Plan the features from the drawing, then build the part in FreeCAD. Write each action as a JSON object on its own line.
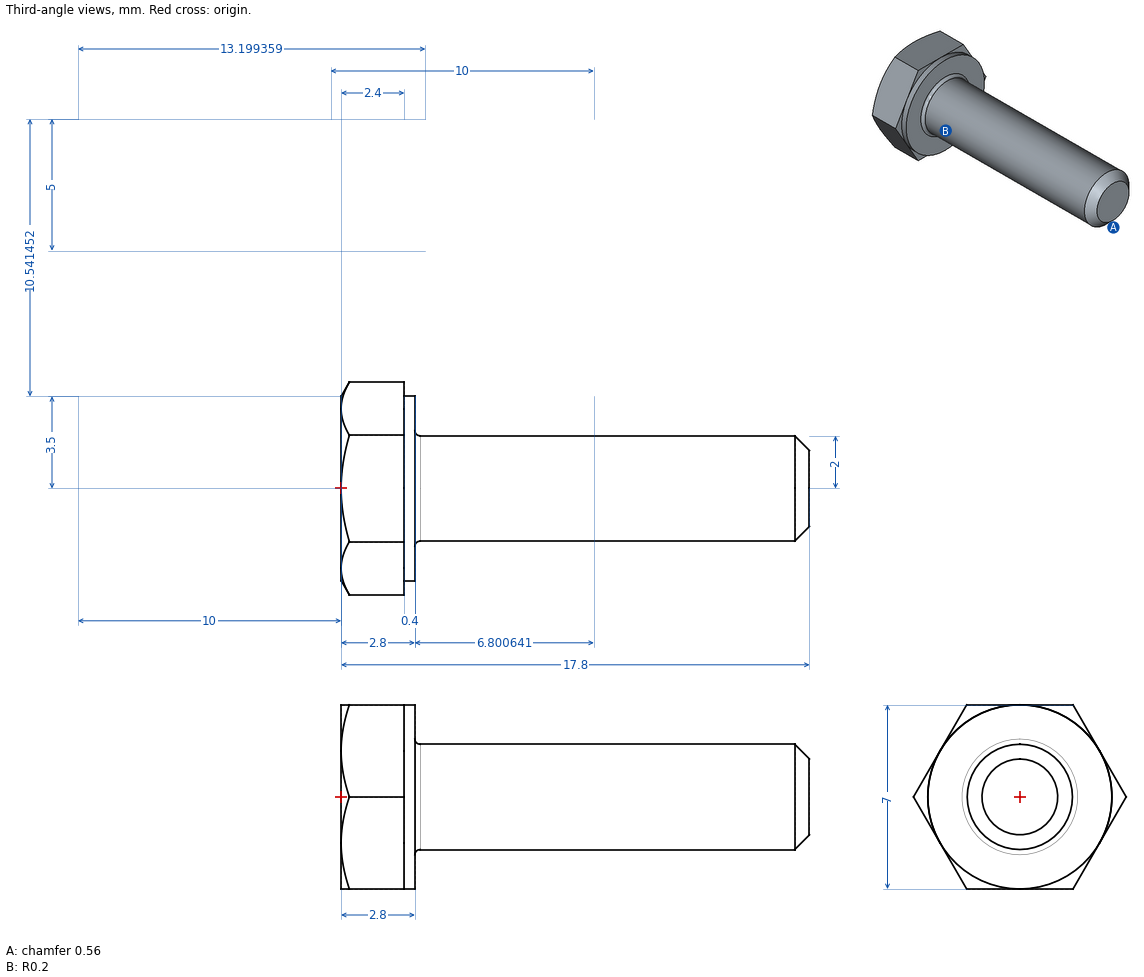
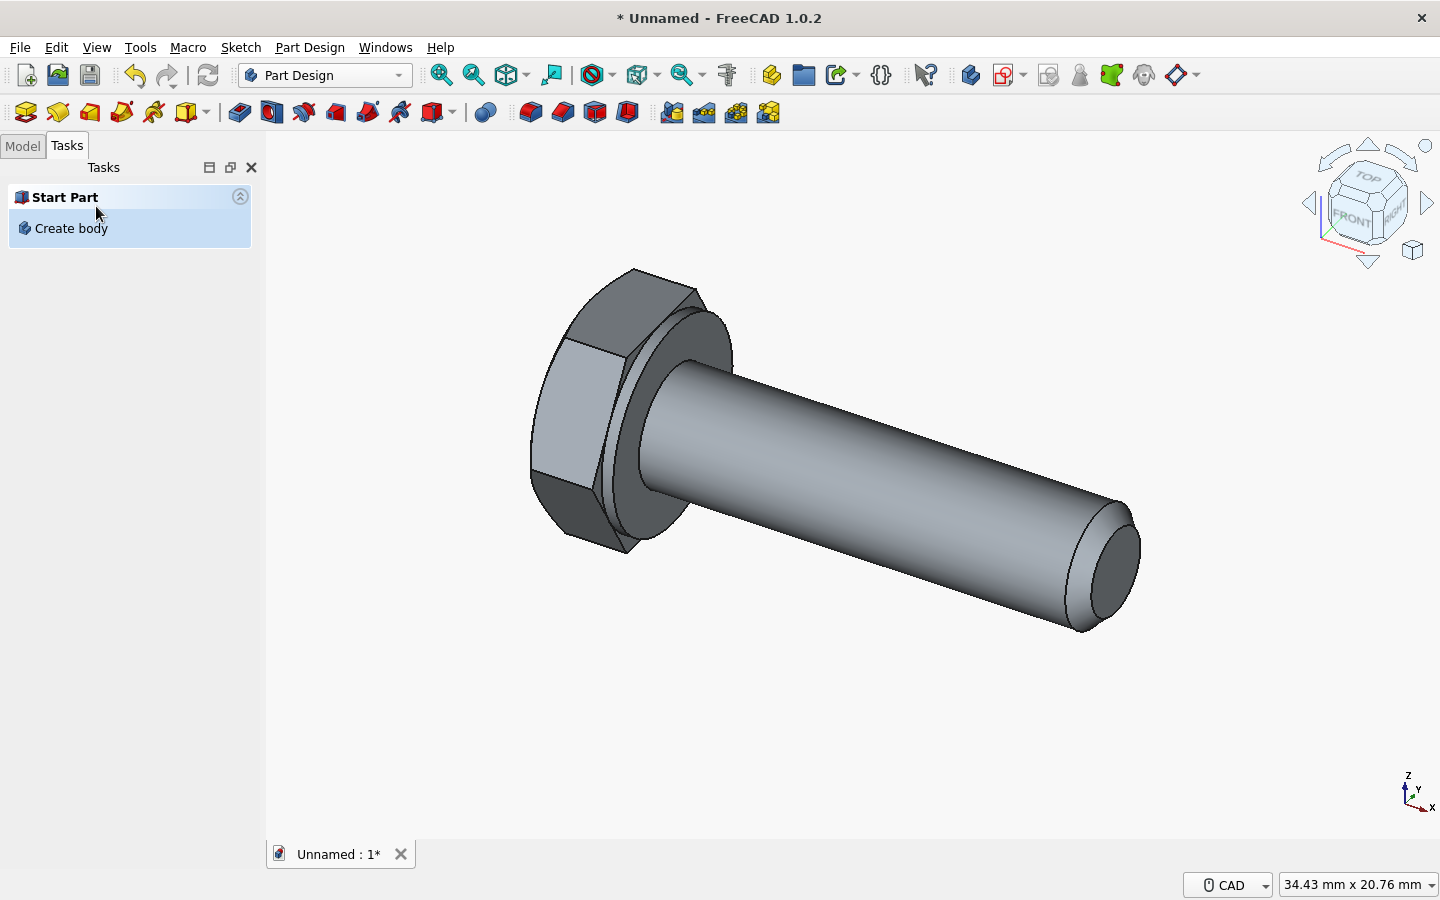
{"action": "key", "text": "0"}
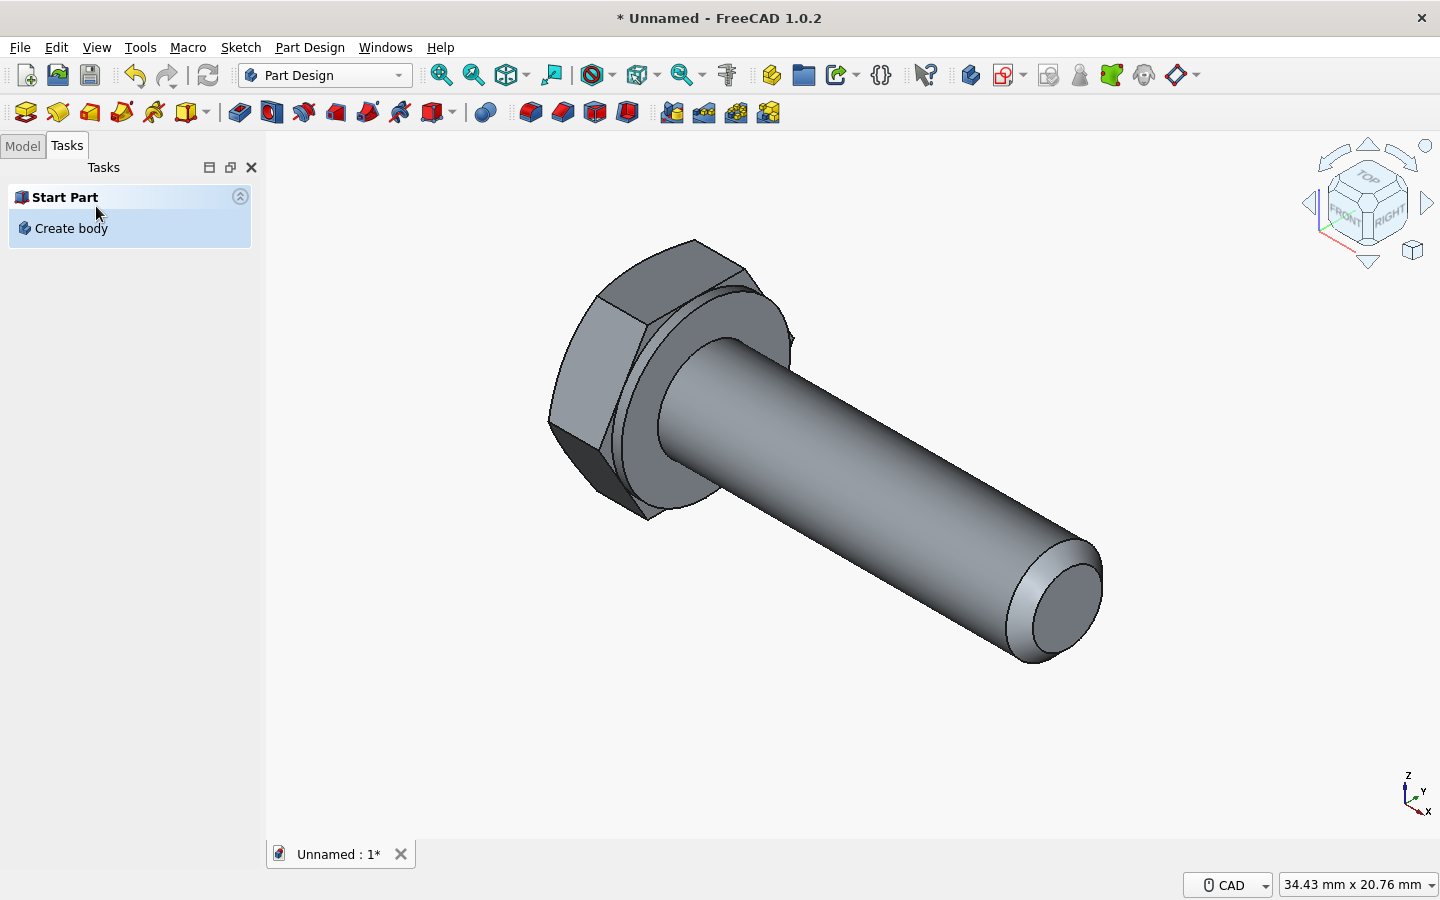
{"action": "key", "text": "2"}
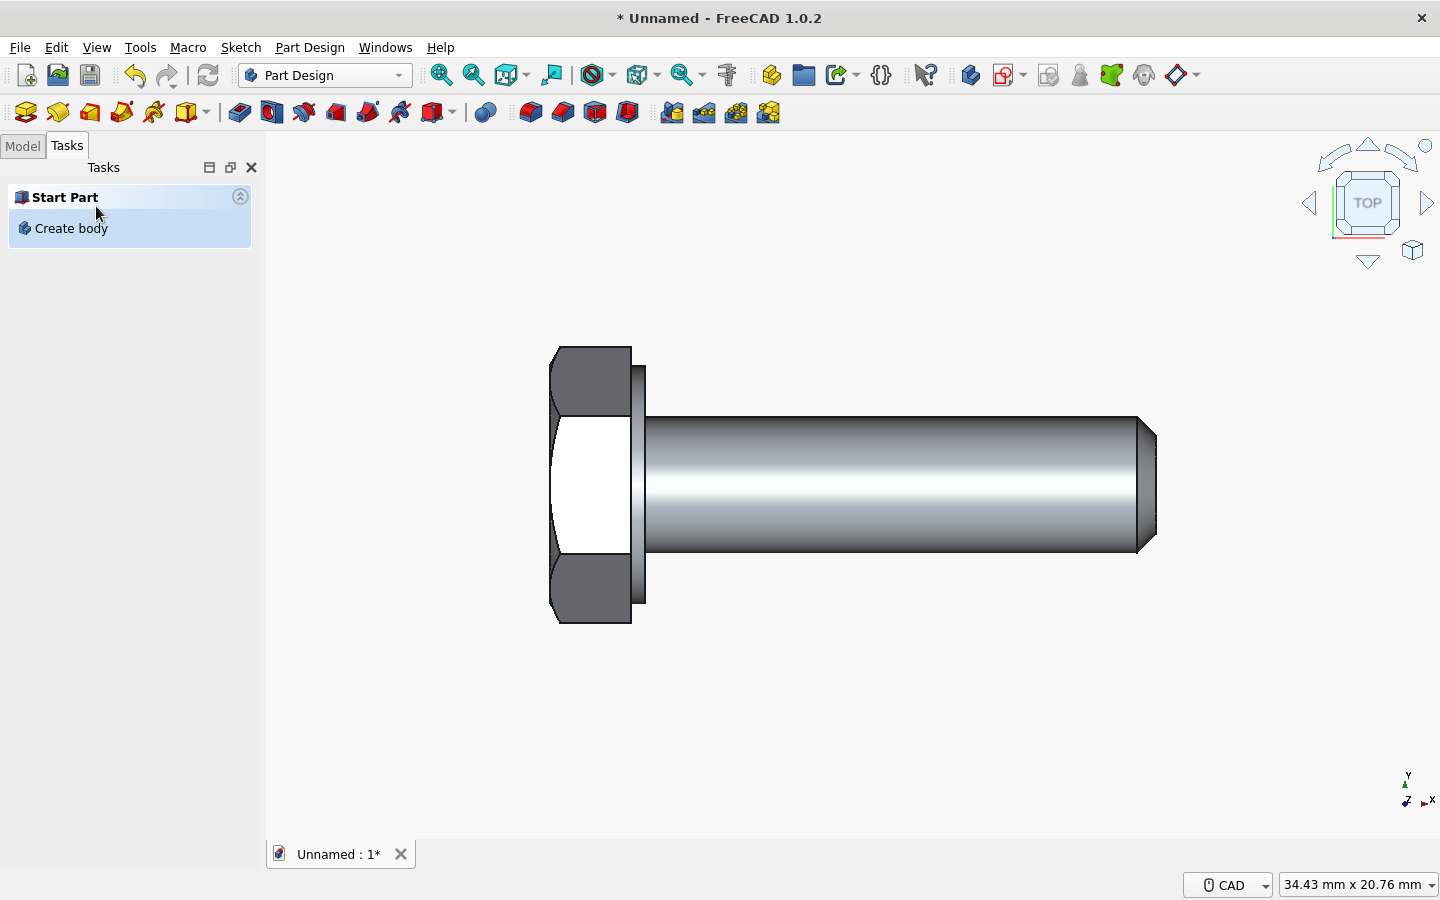
{"action": "key", "text": "1"}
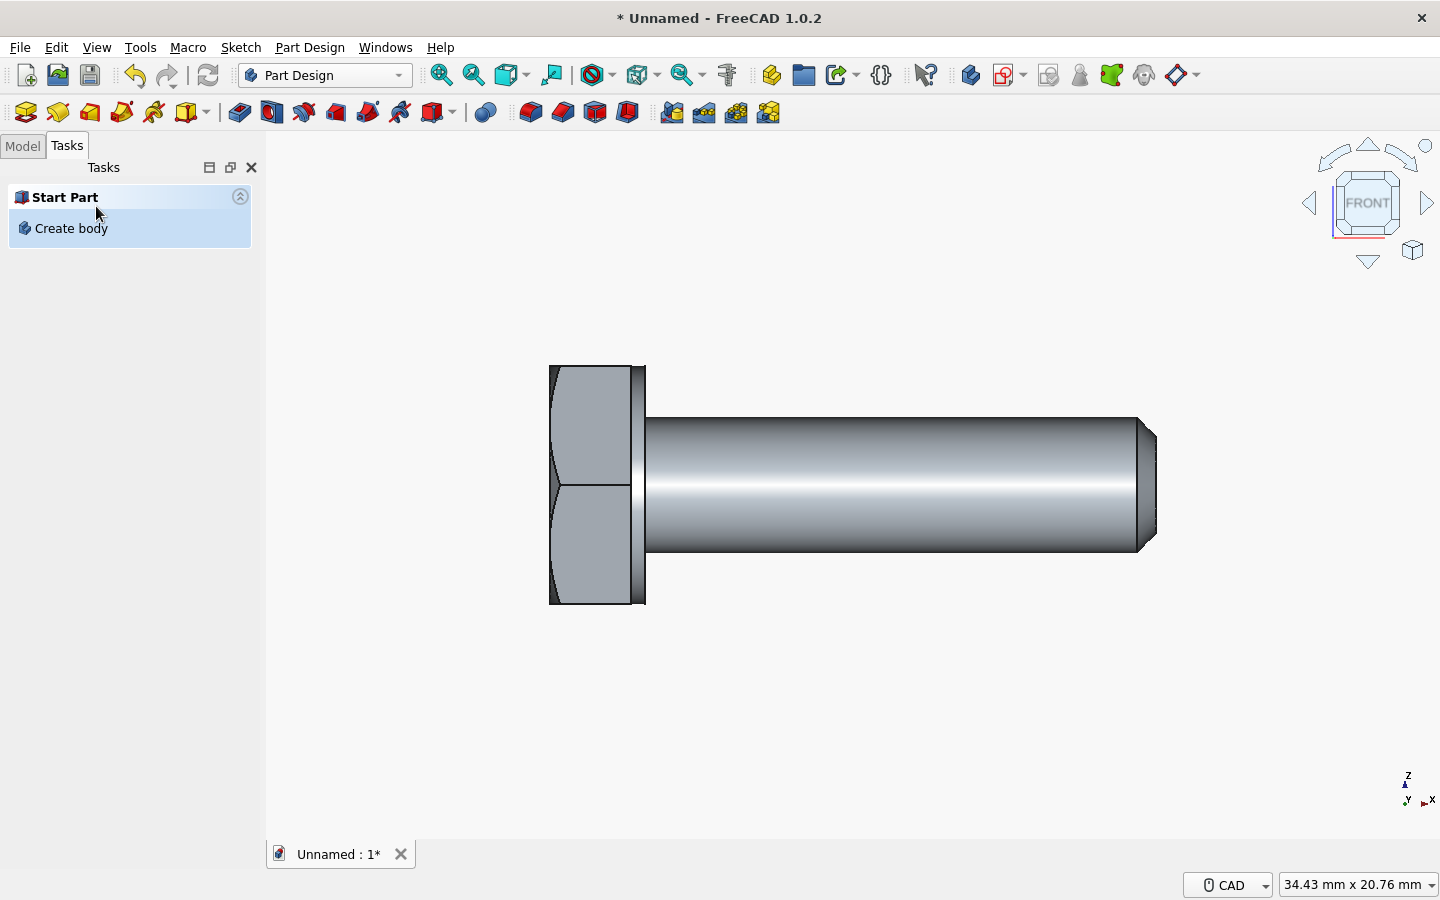
{"action": "key", "text": "3"}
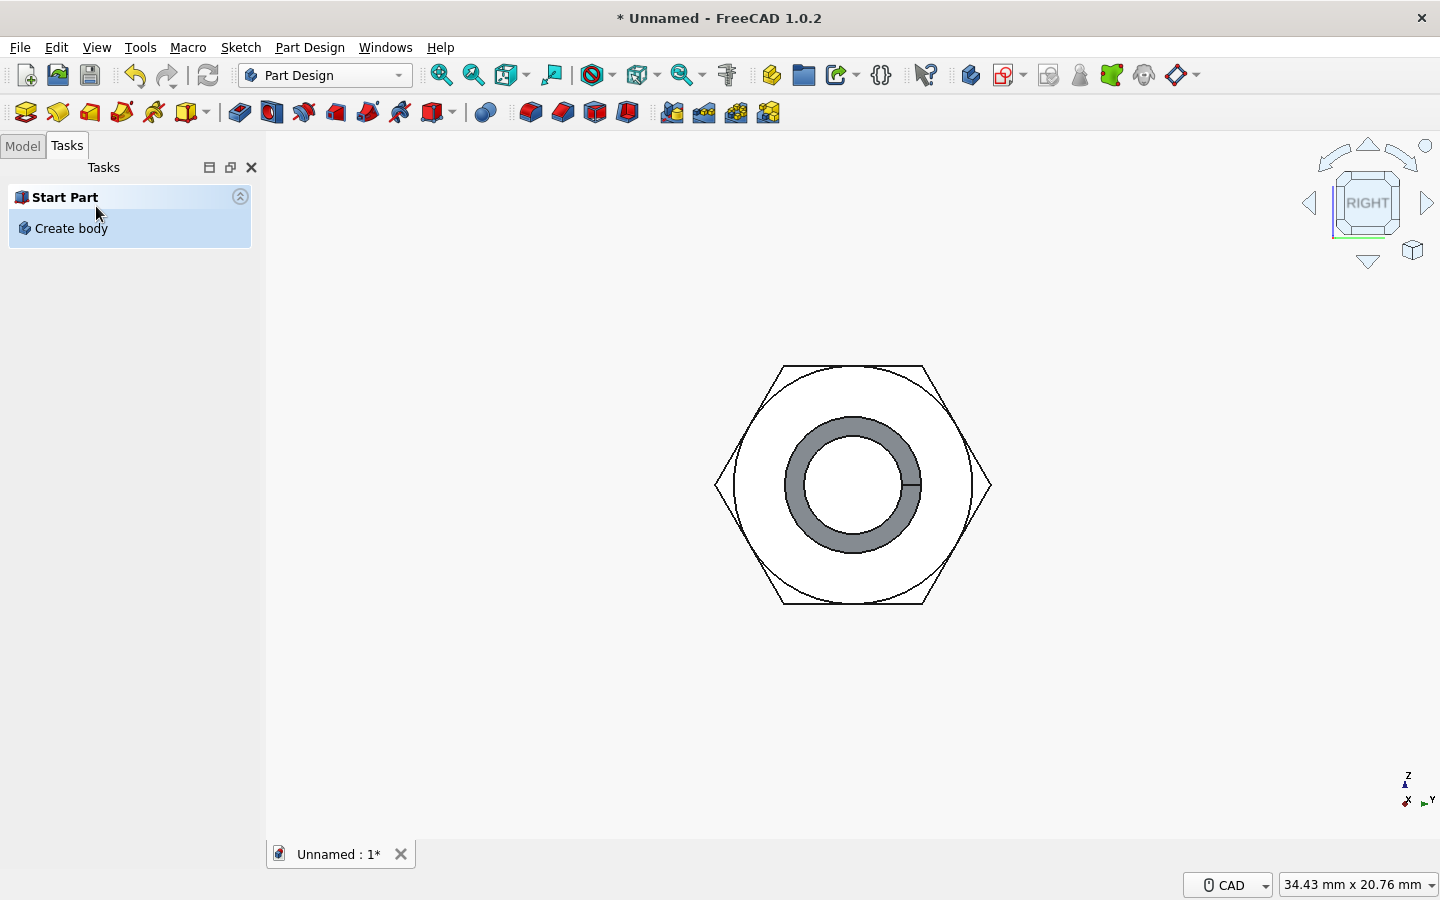
{"action": "key", "text": "v f"}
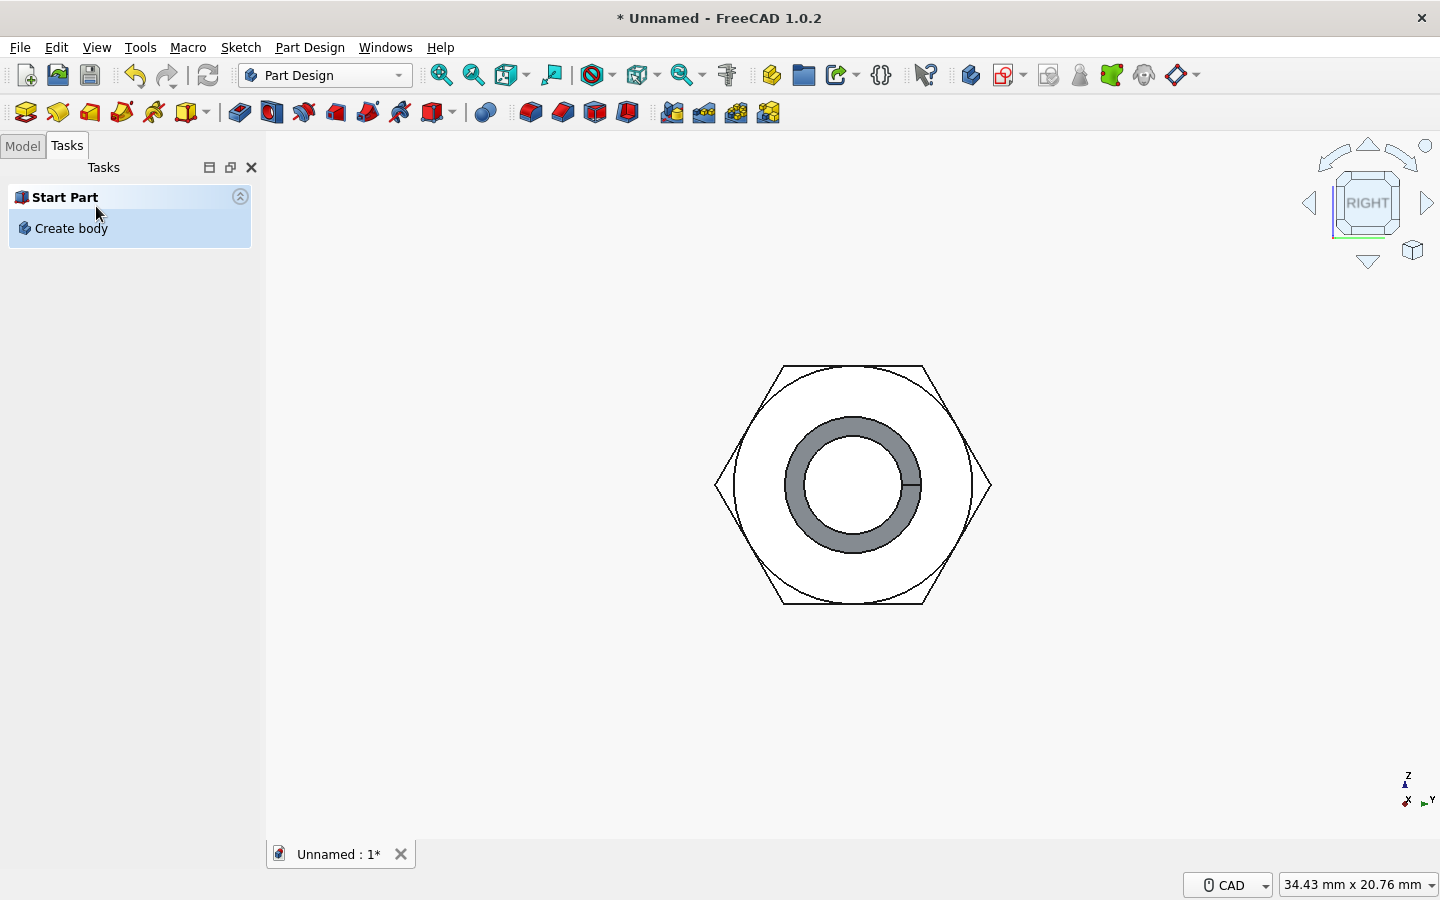
{"action": "key", "text": "5"}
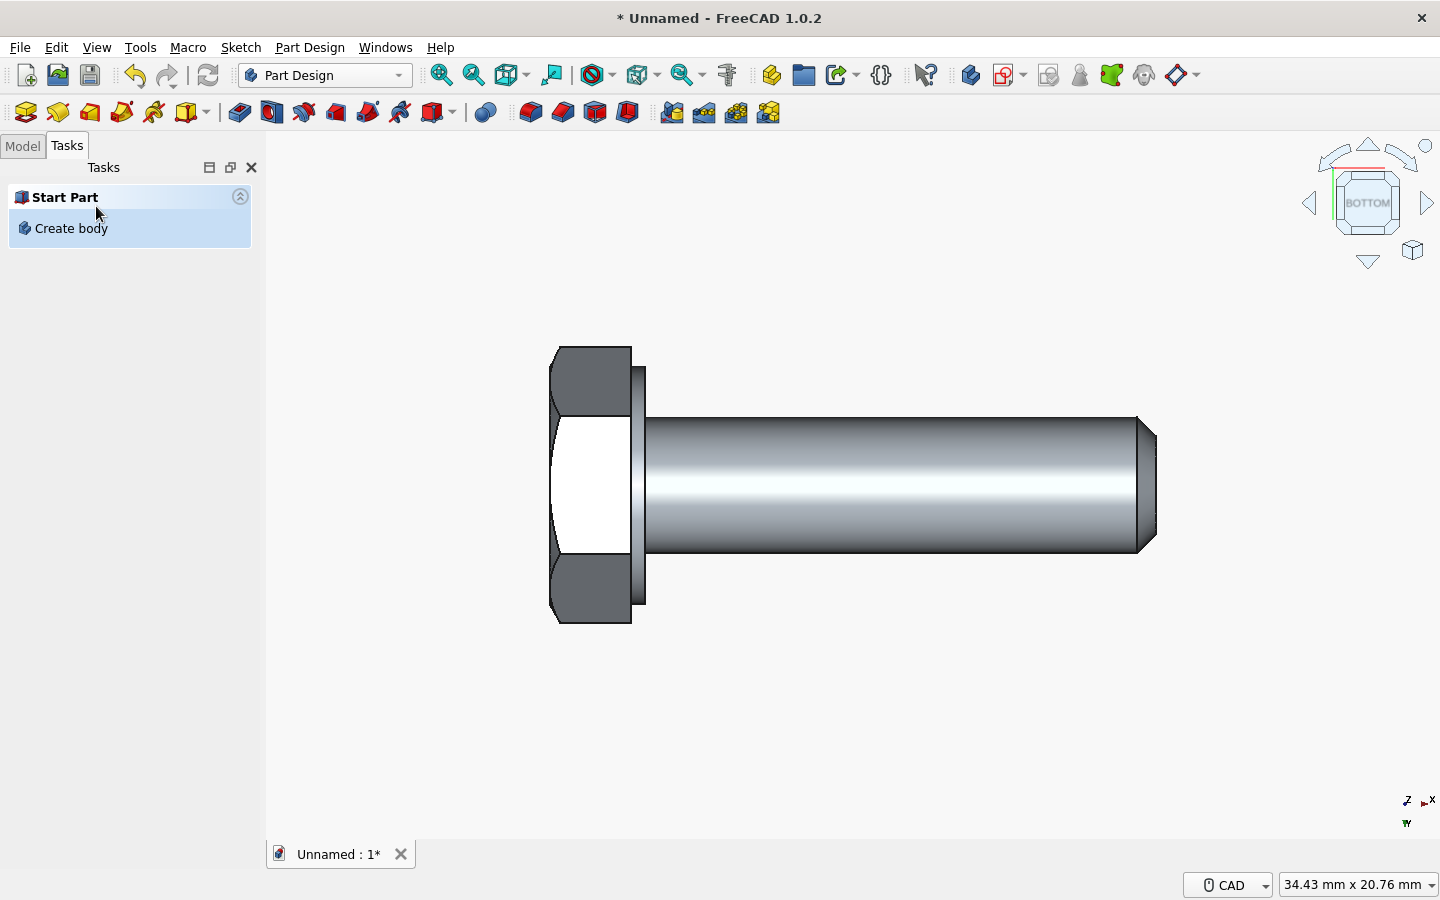
{"action": "key", "text": "4"}